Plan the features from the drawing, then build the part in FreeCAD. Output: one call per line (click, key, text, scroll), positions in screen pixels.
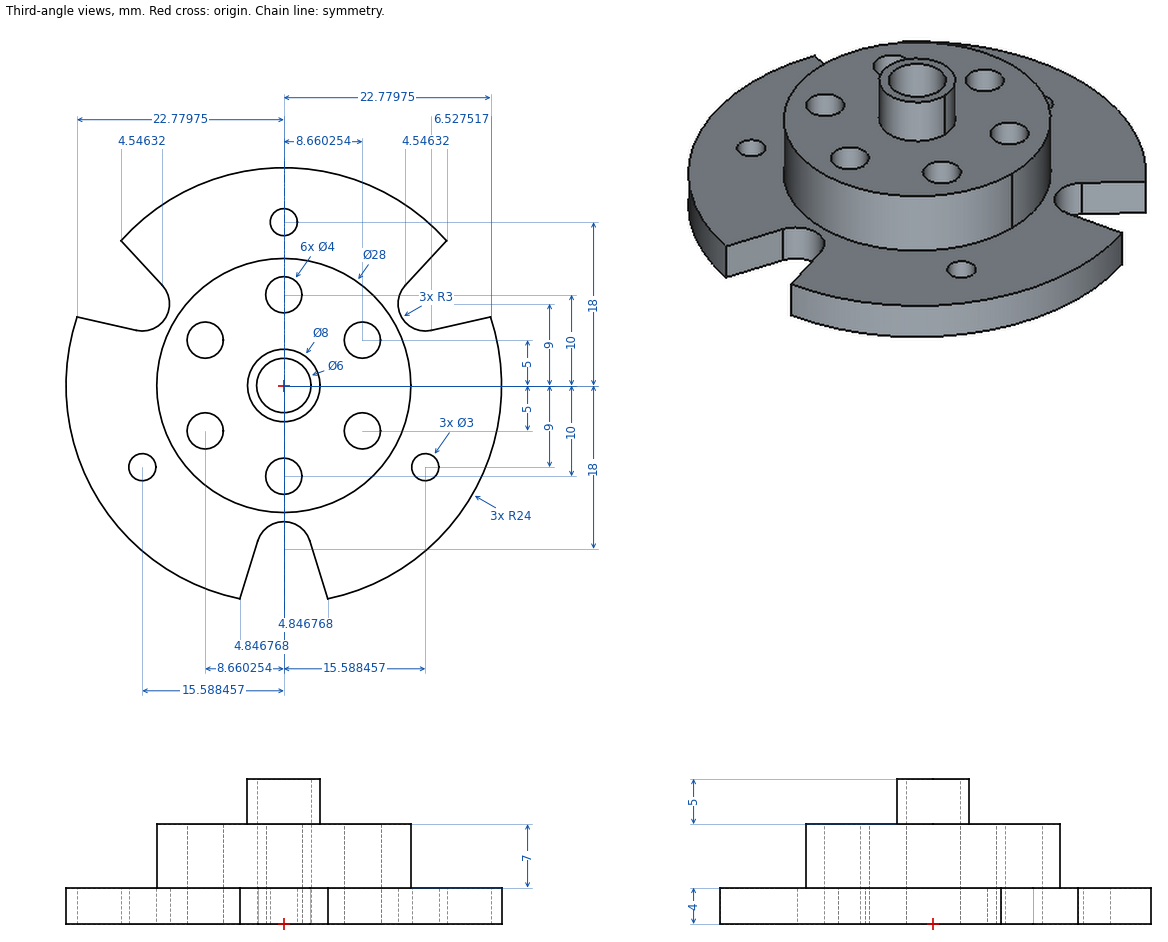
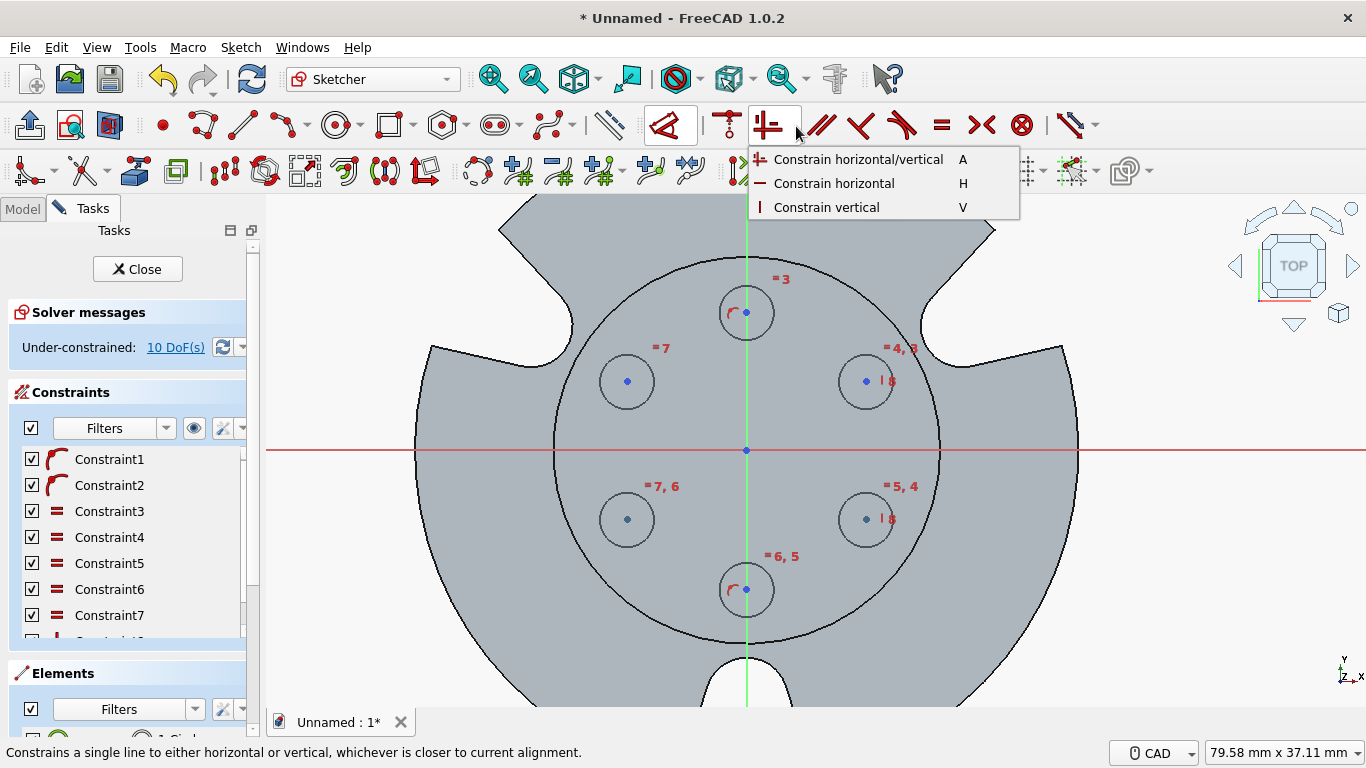
click(884, 183)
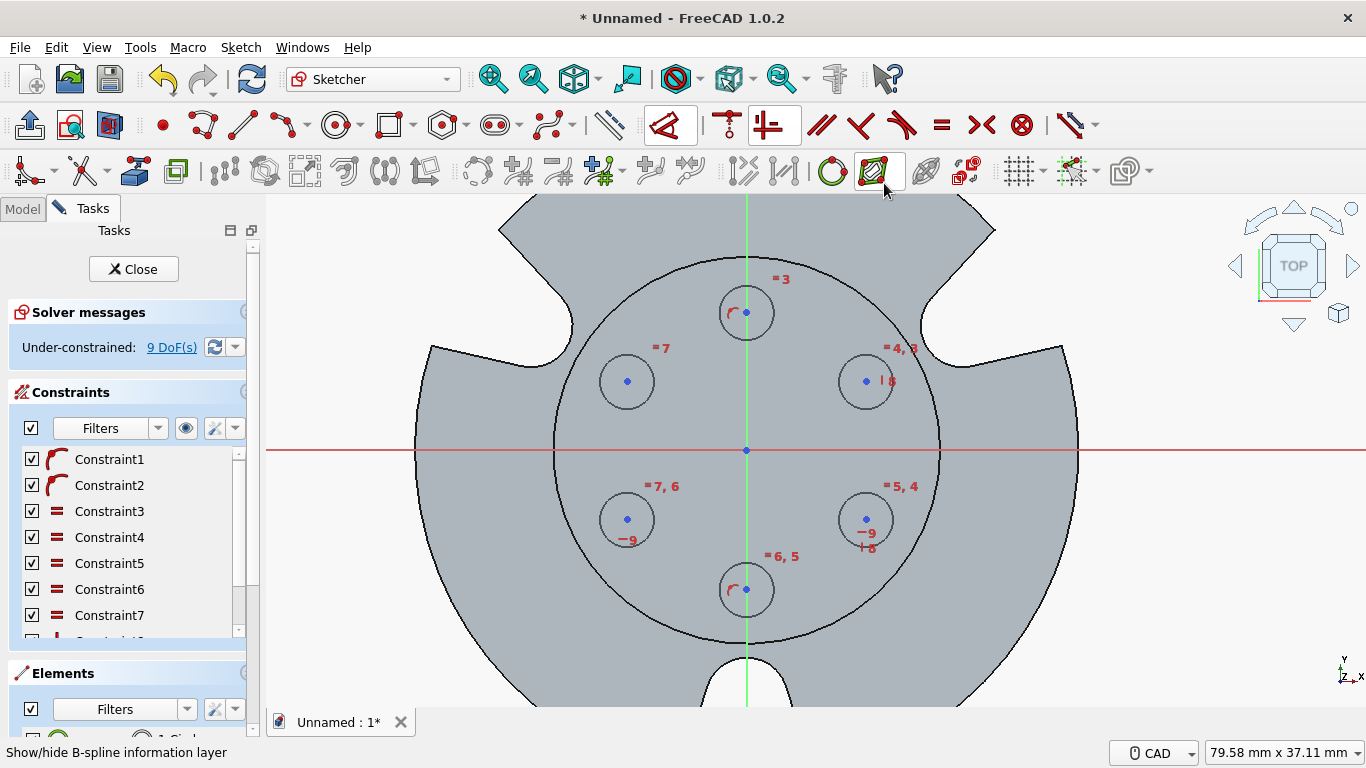
click(627, 520)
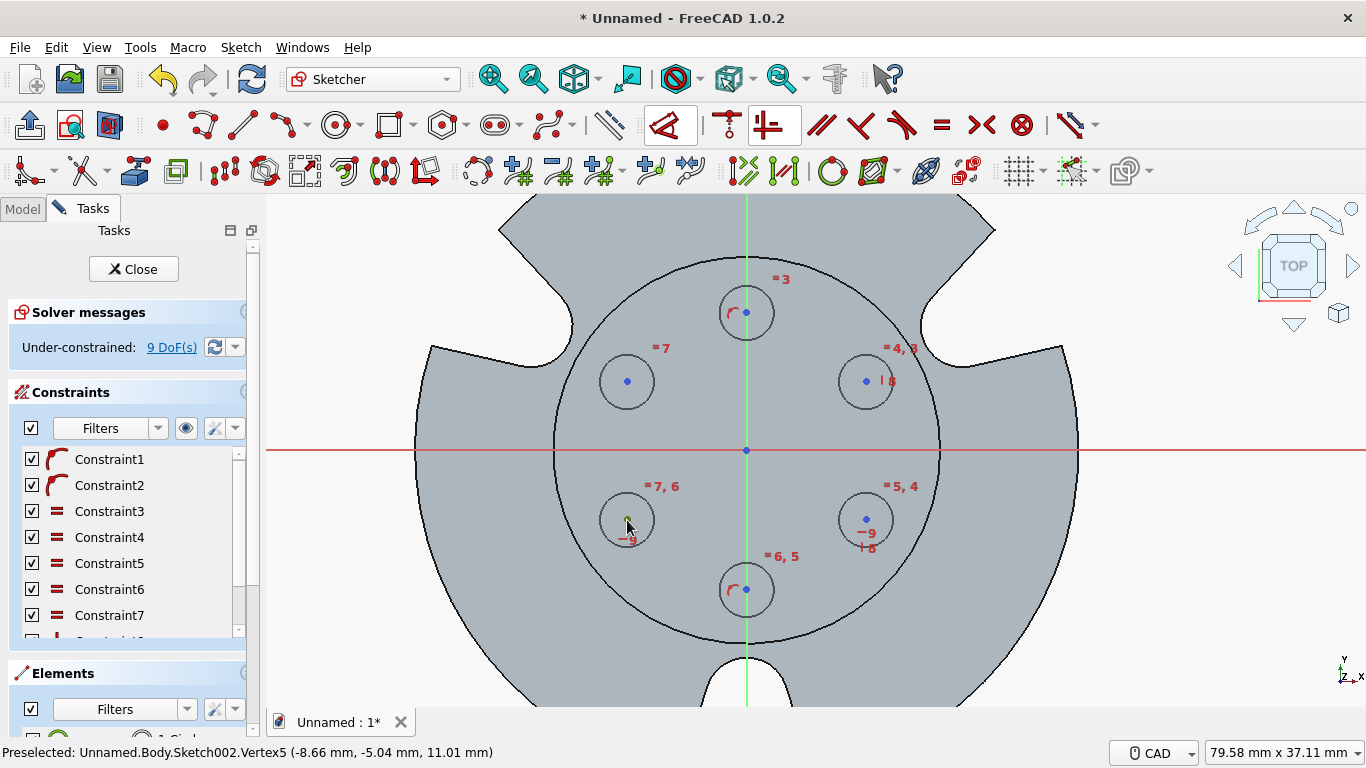
click(627, 382)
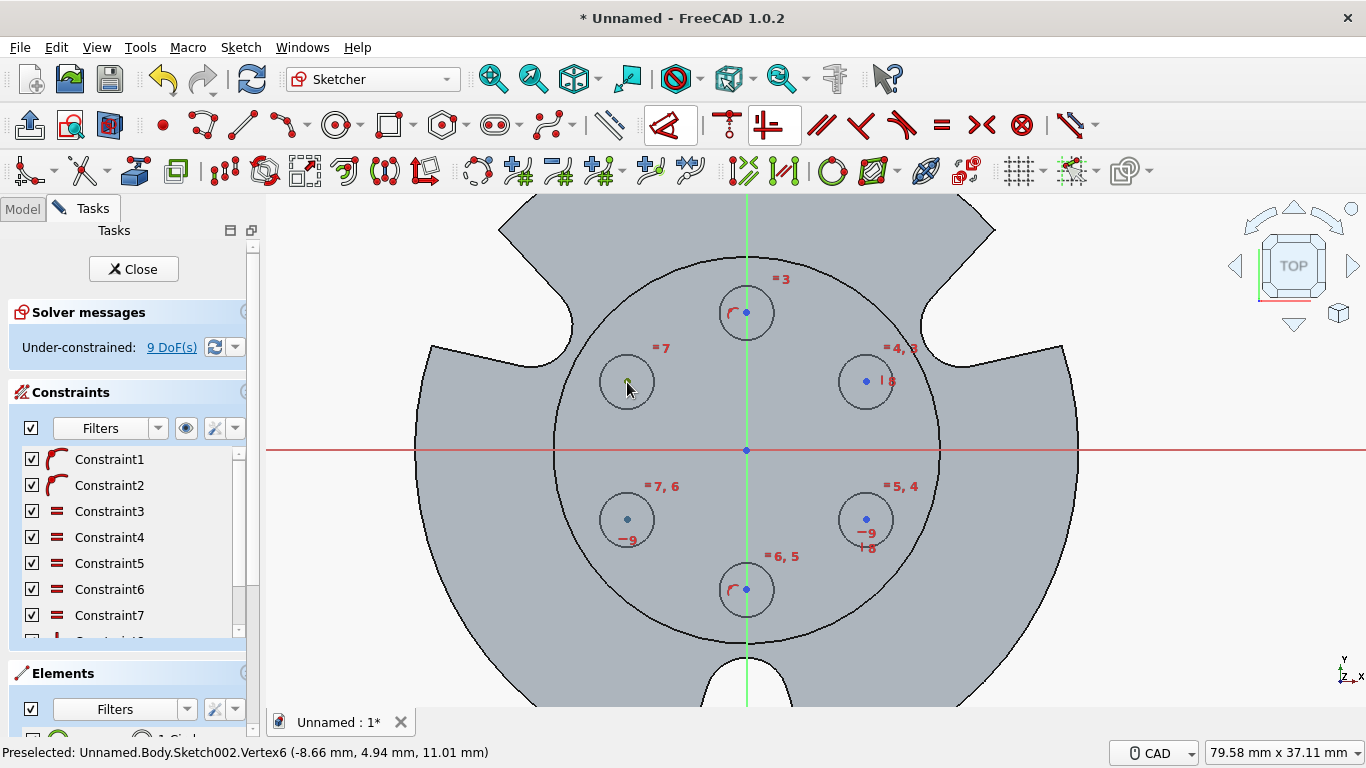
click(796, 126)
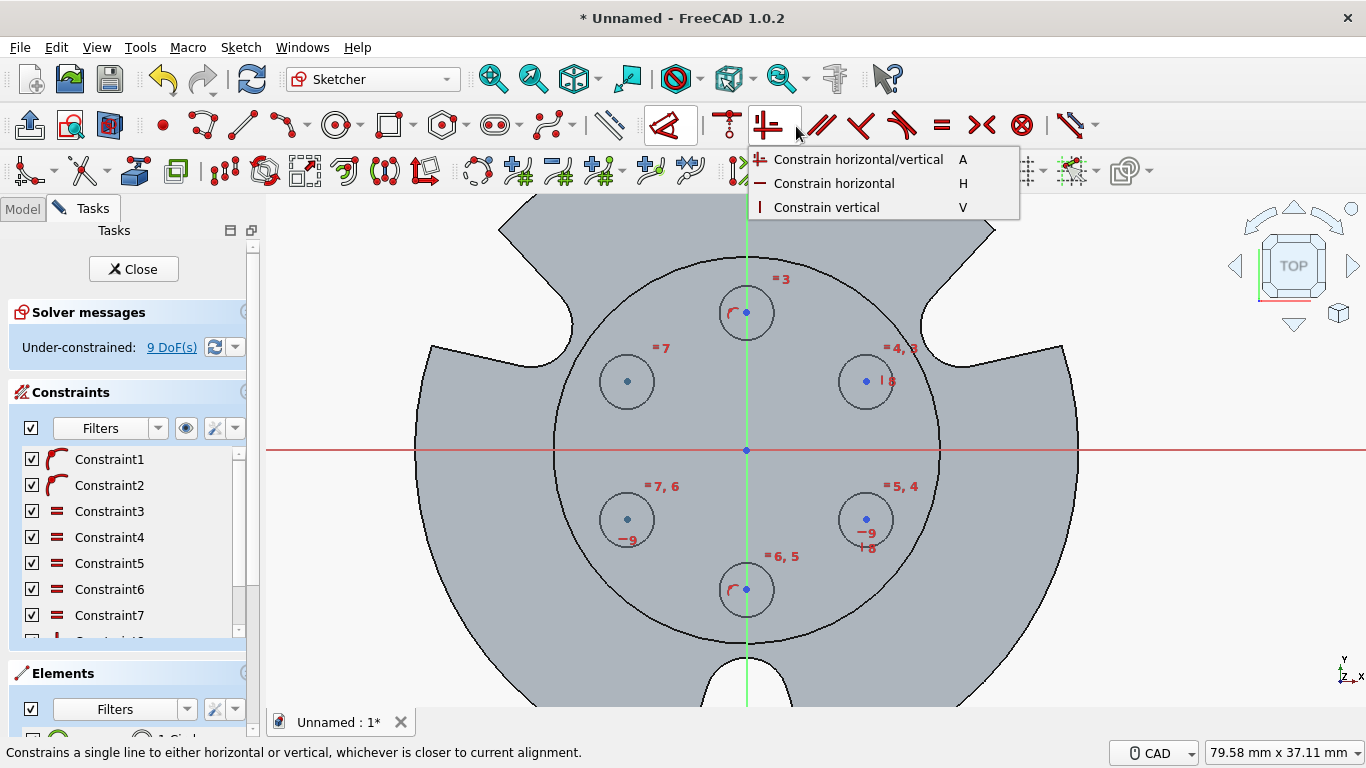
click(884, 207)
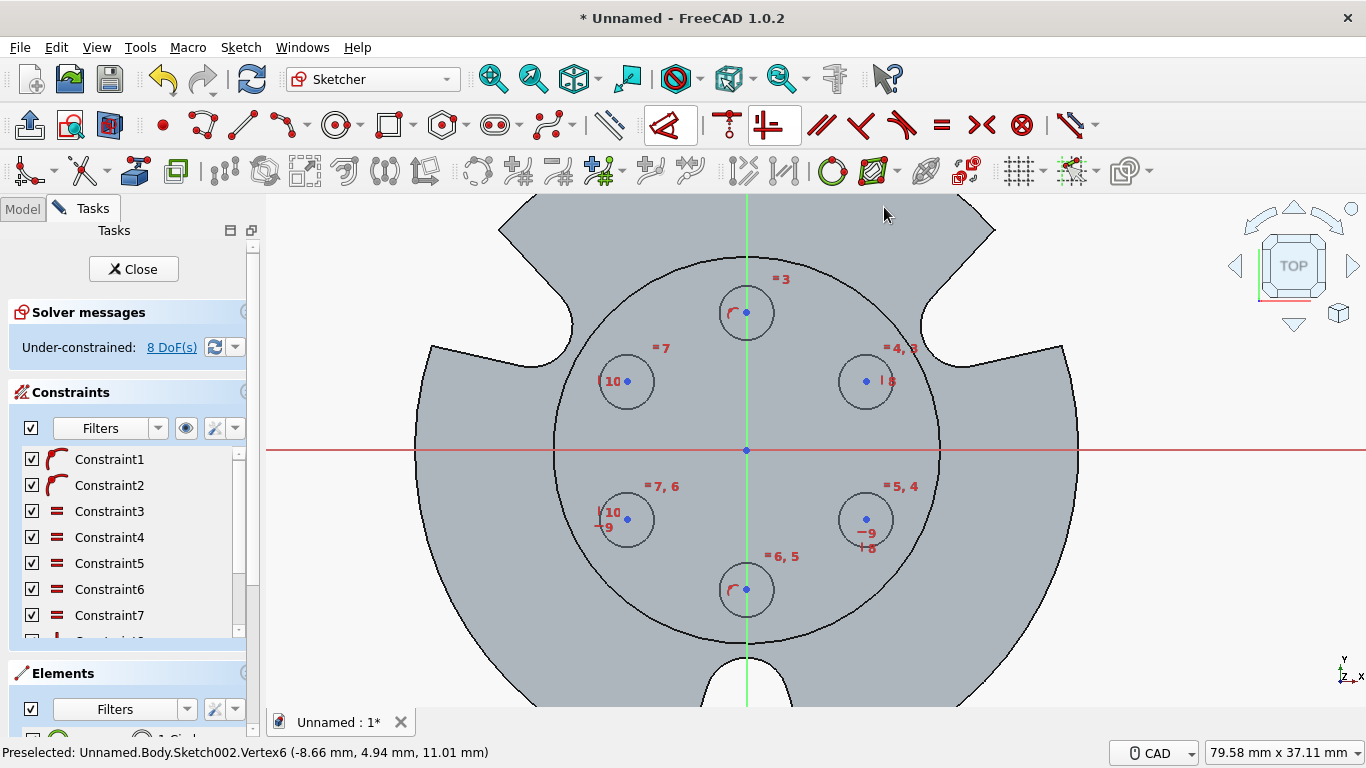
click(866, 382)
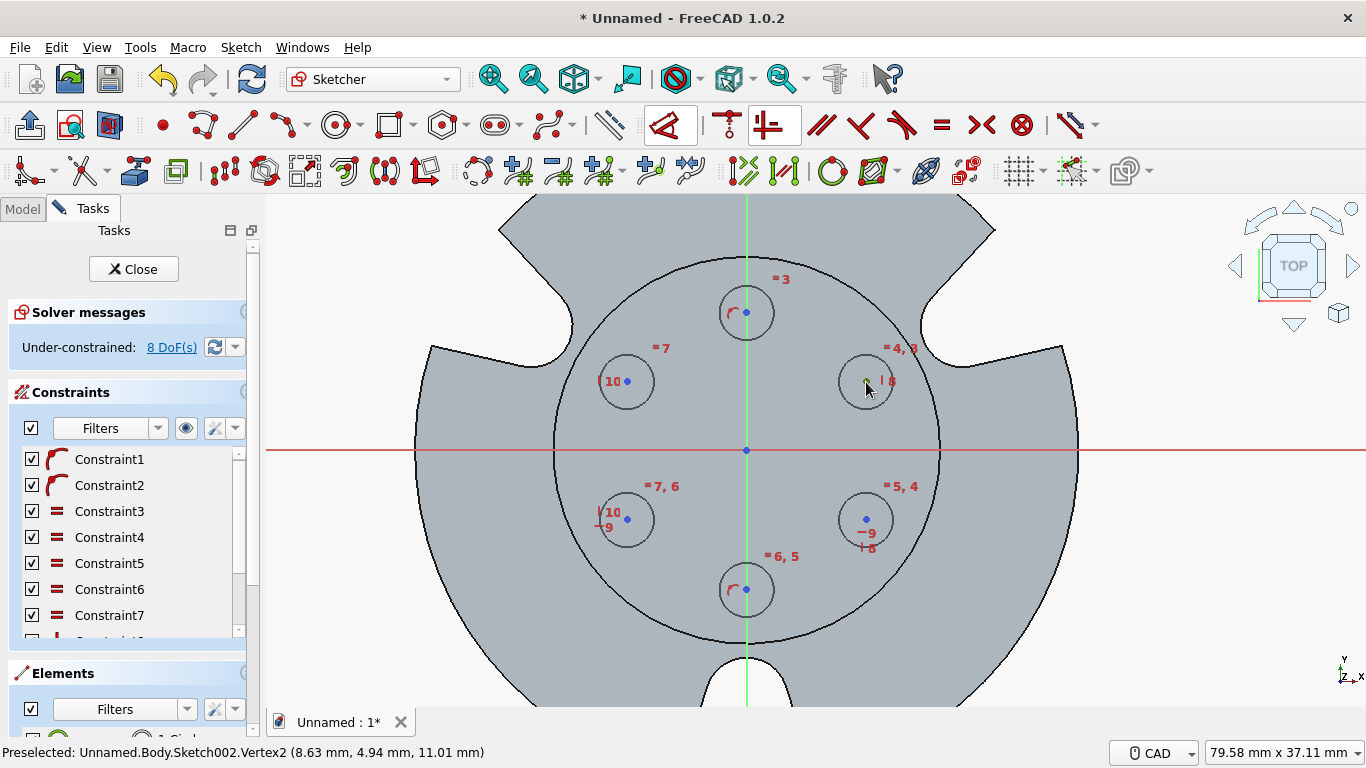
click(627, 382)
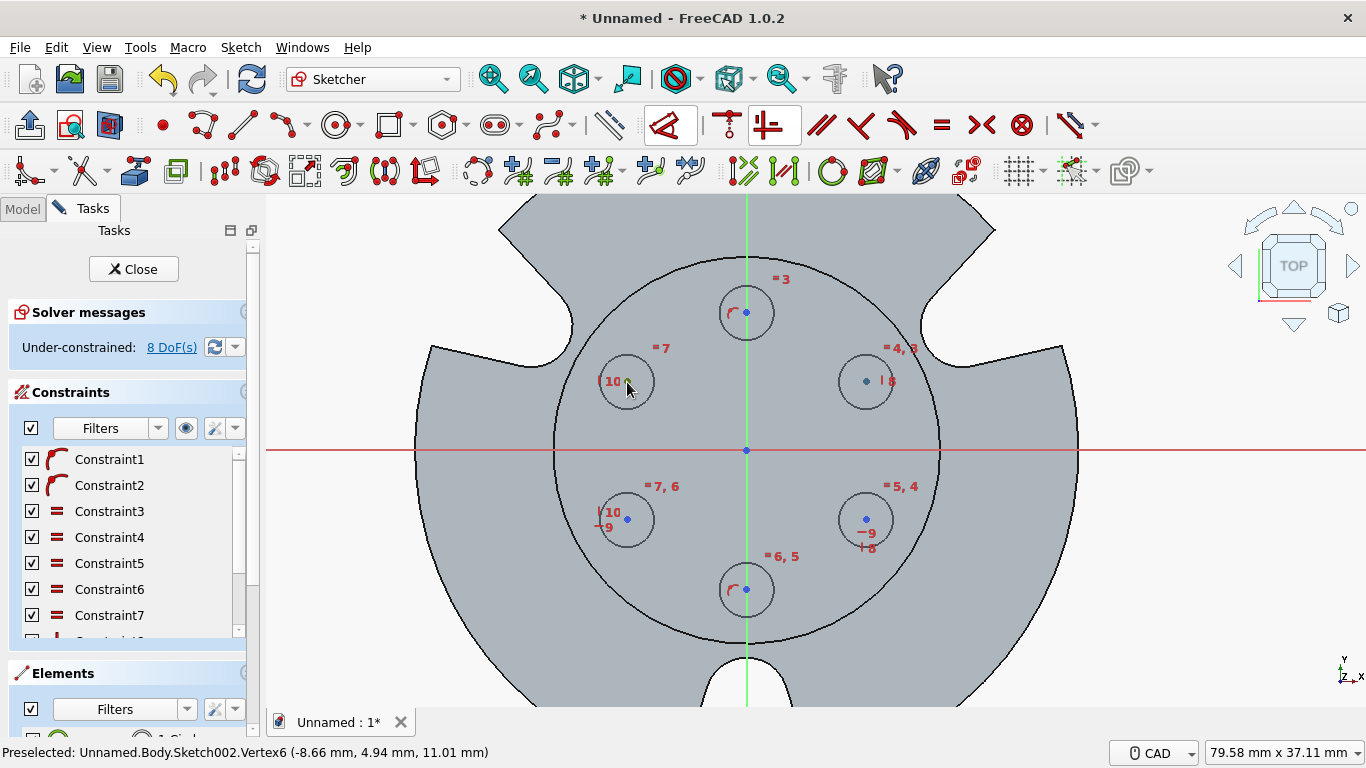
key(h)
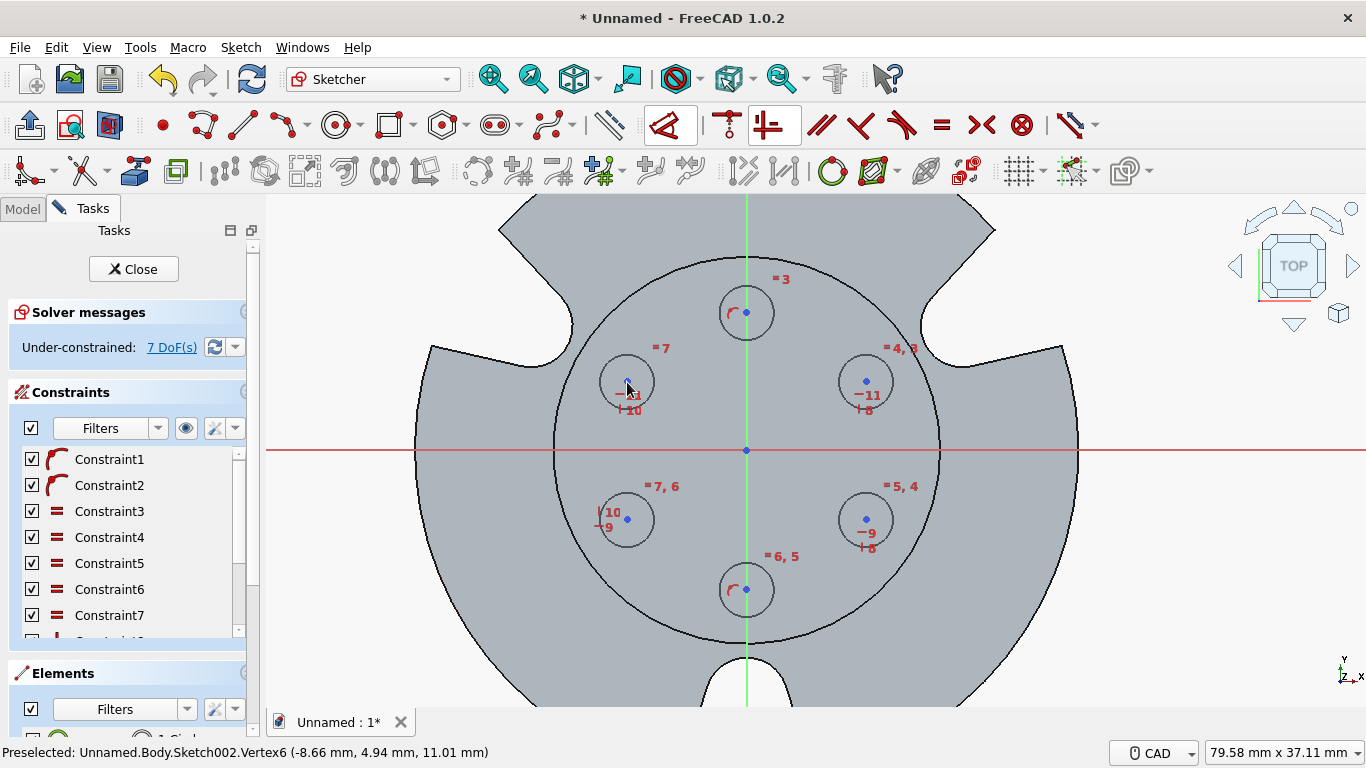
click(664, 126)